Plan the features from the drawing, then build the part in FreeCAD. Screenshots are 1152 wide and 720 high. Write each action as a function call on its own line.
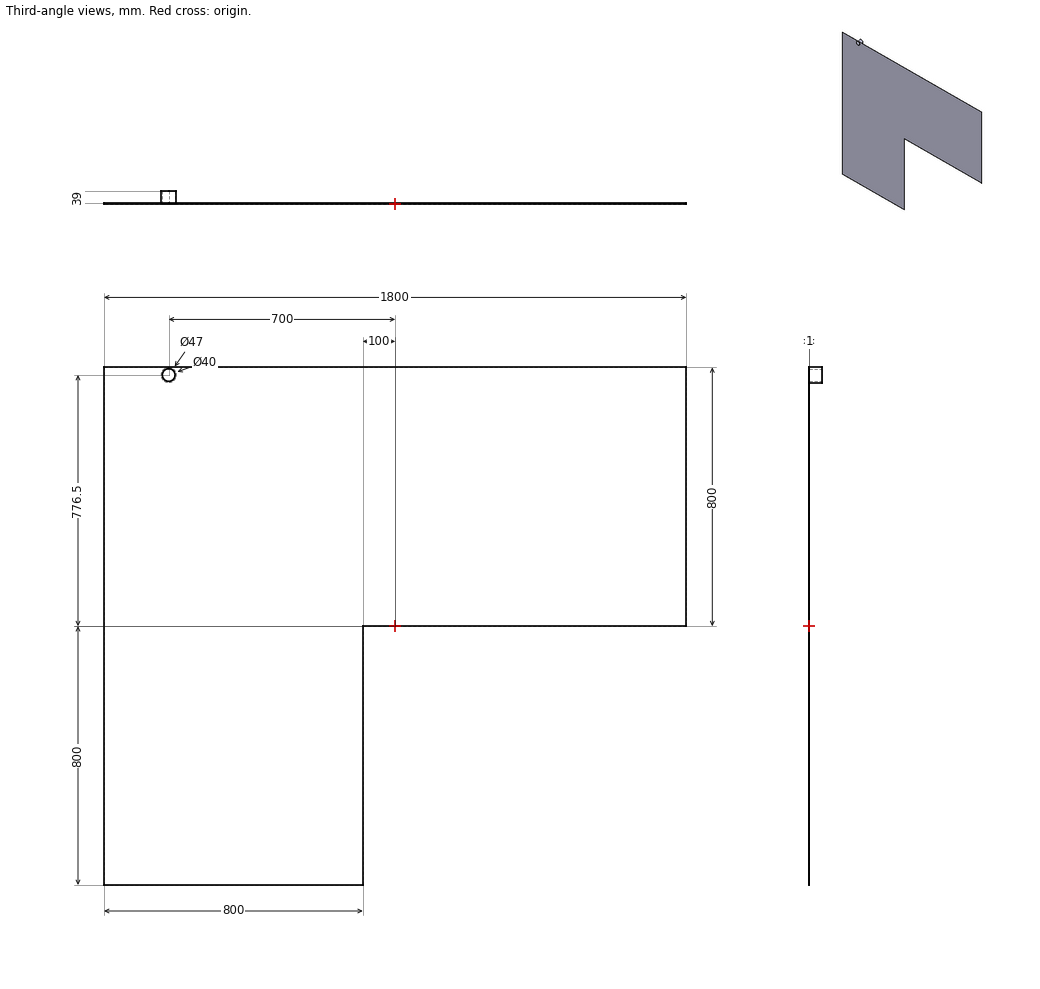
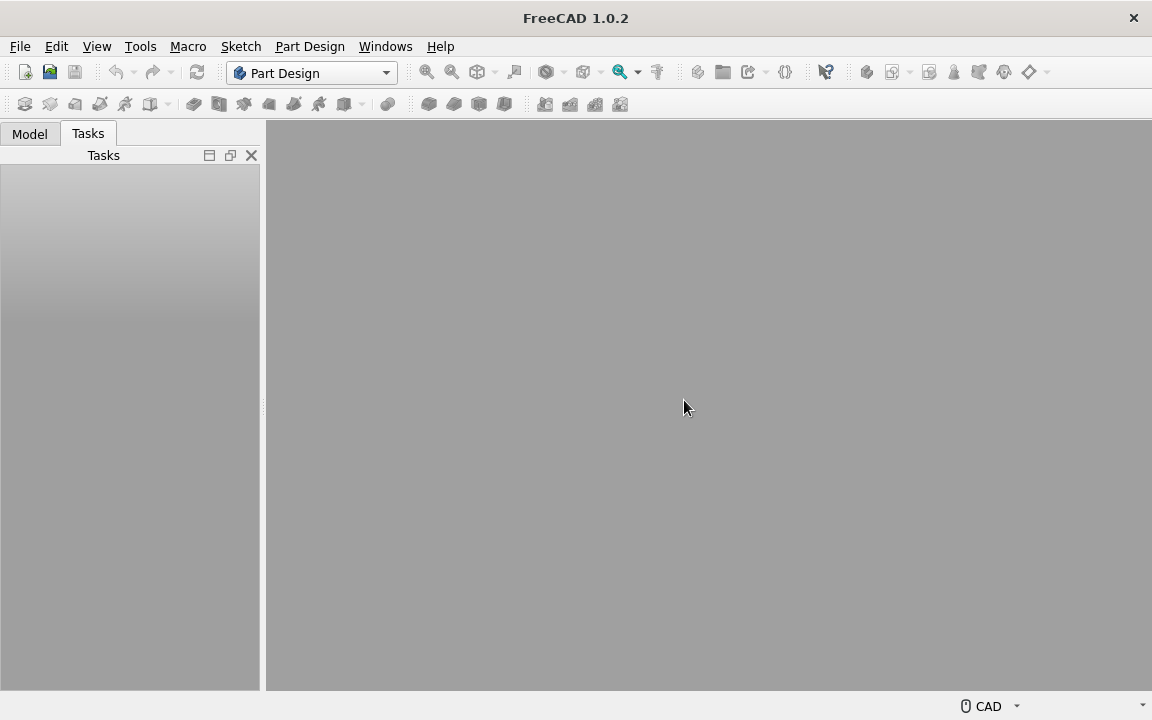
click(25, 72)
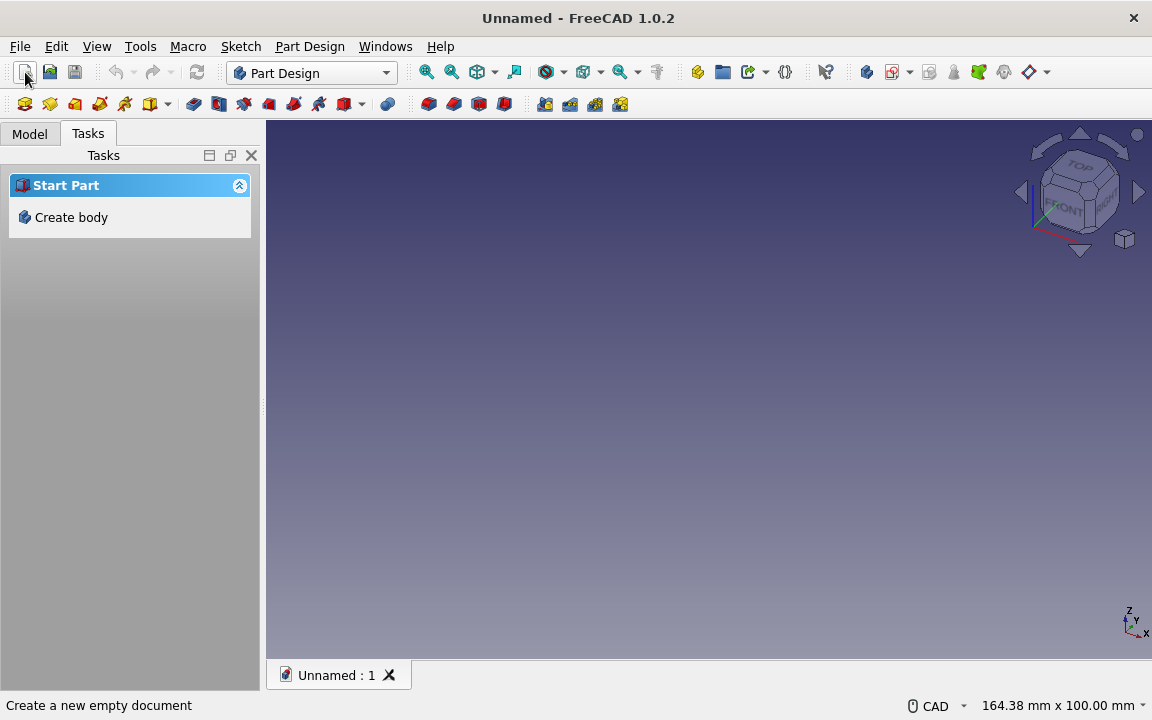
click(892, 72)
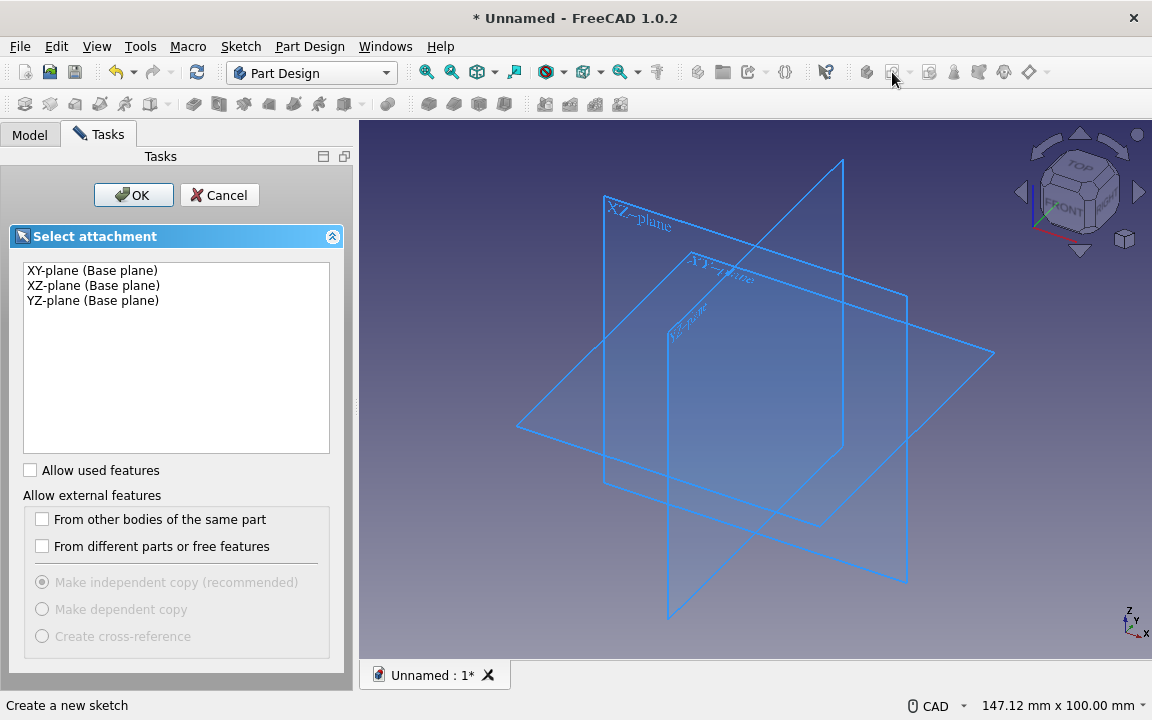
click(84, 286)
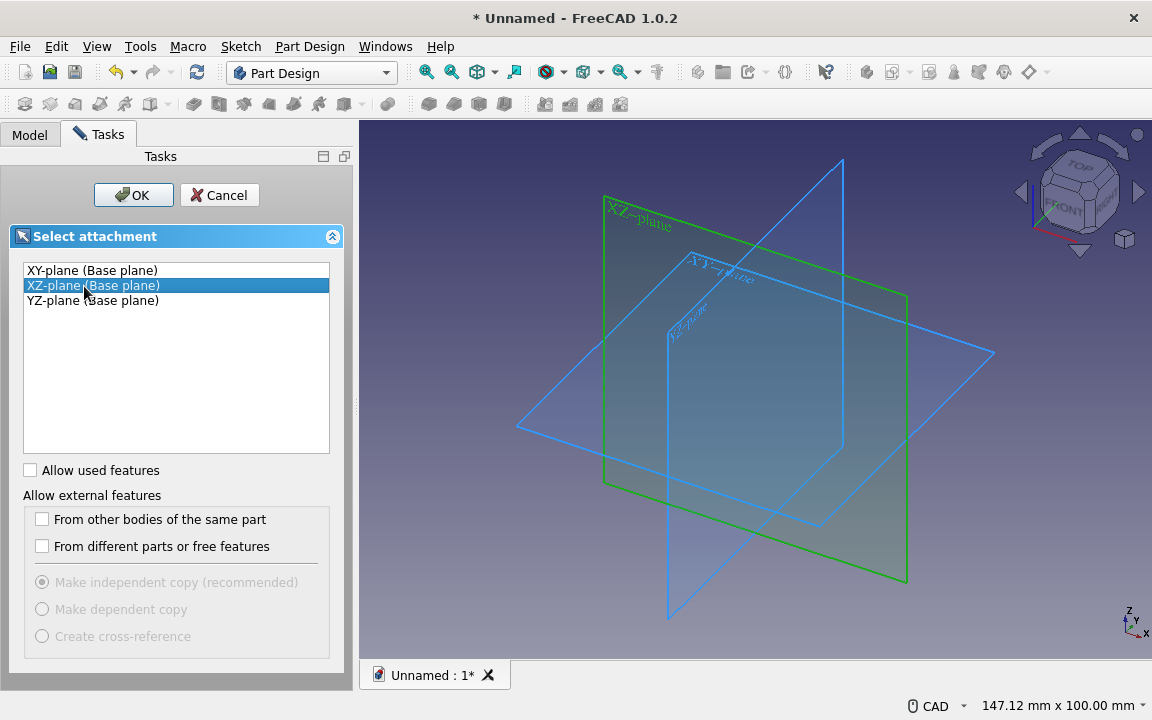
click(134, 195)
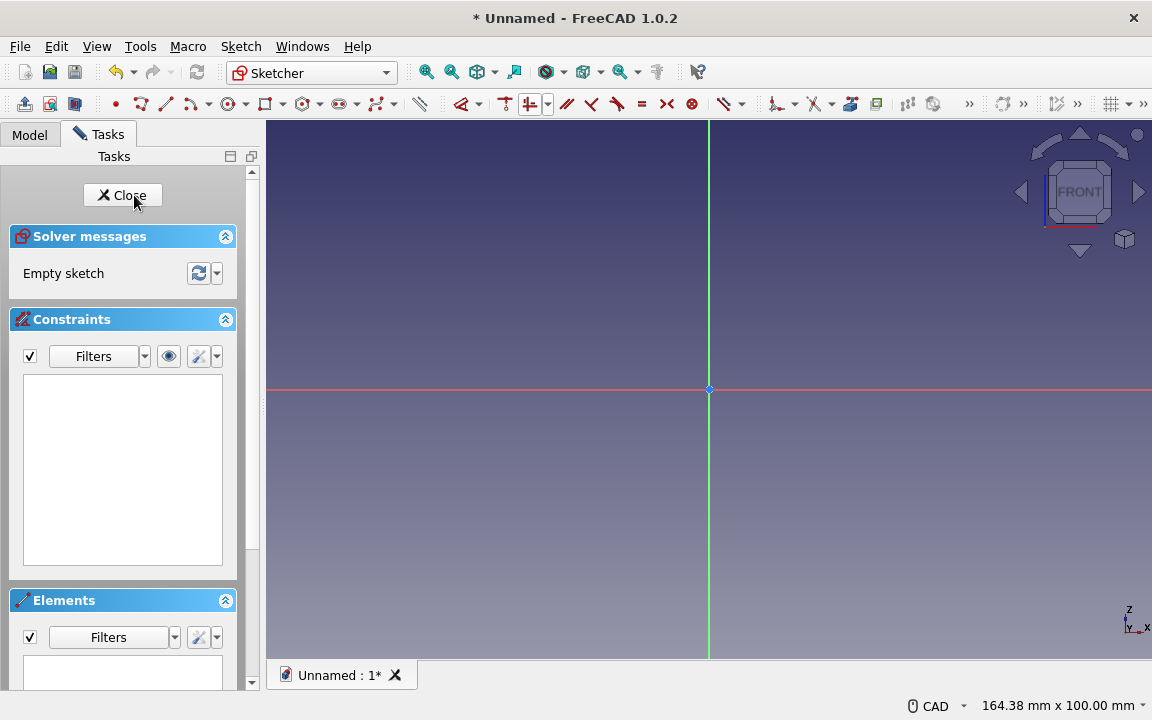
scroll(637, 390, down, 15)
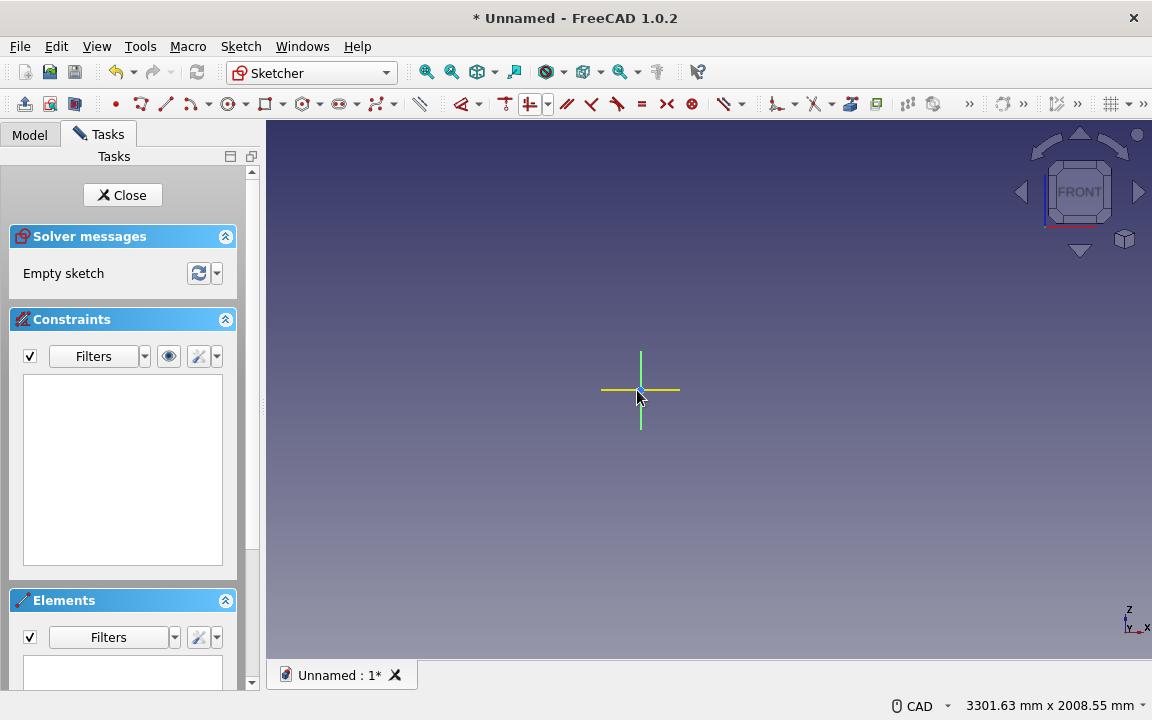
click(141, 104)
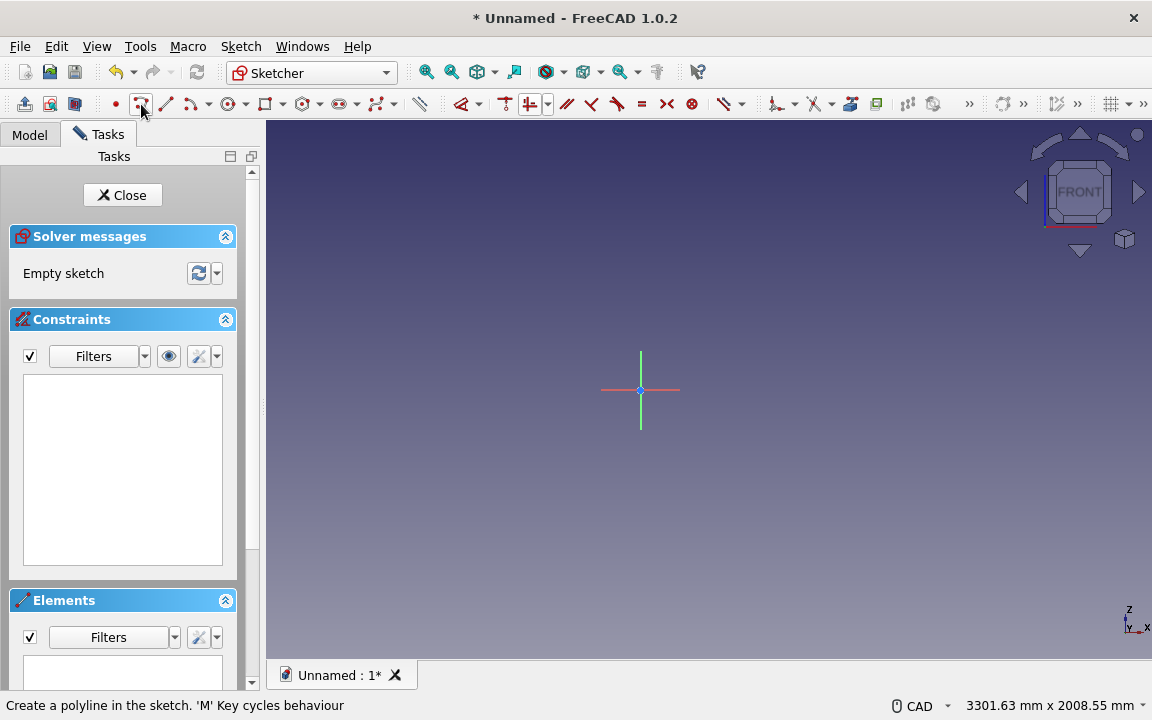
click(614, 390)
click(614, 605)
click(399, 605)
click(399, 176)
click(883, 176)
click(883, 381)
click(614, 390)
key(Escape)
key(Escape)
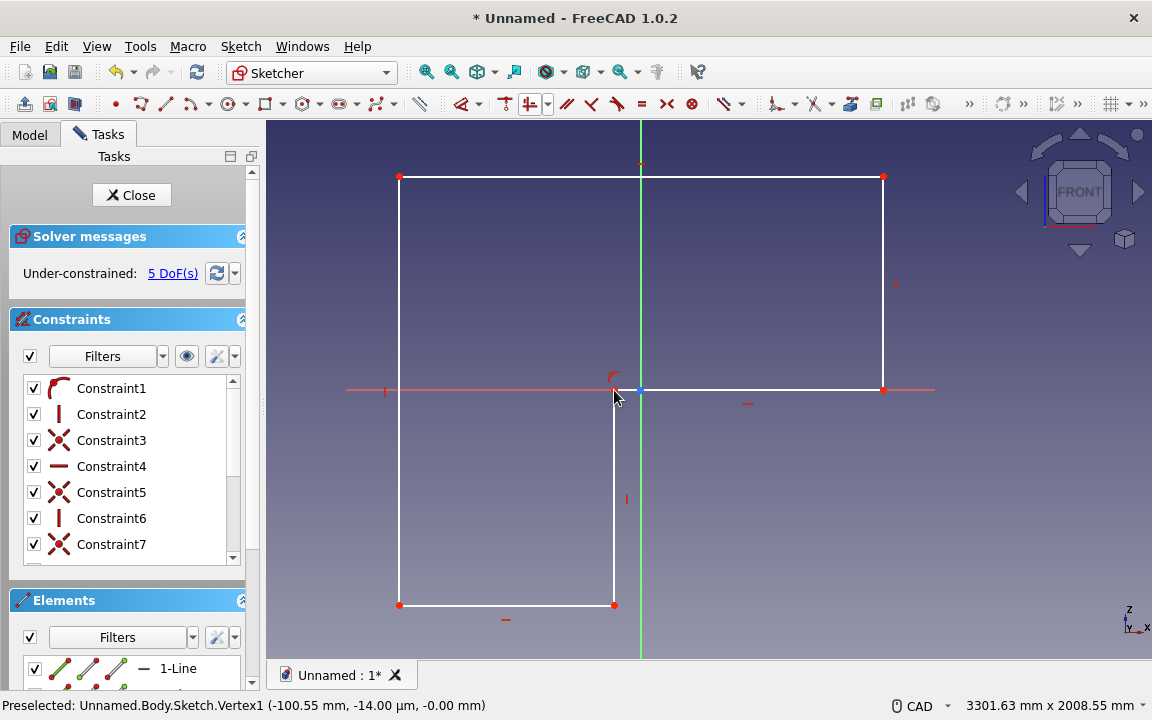
click(614, 455)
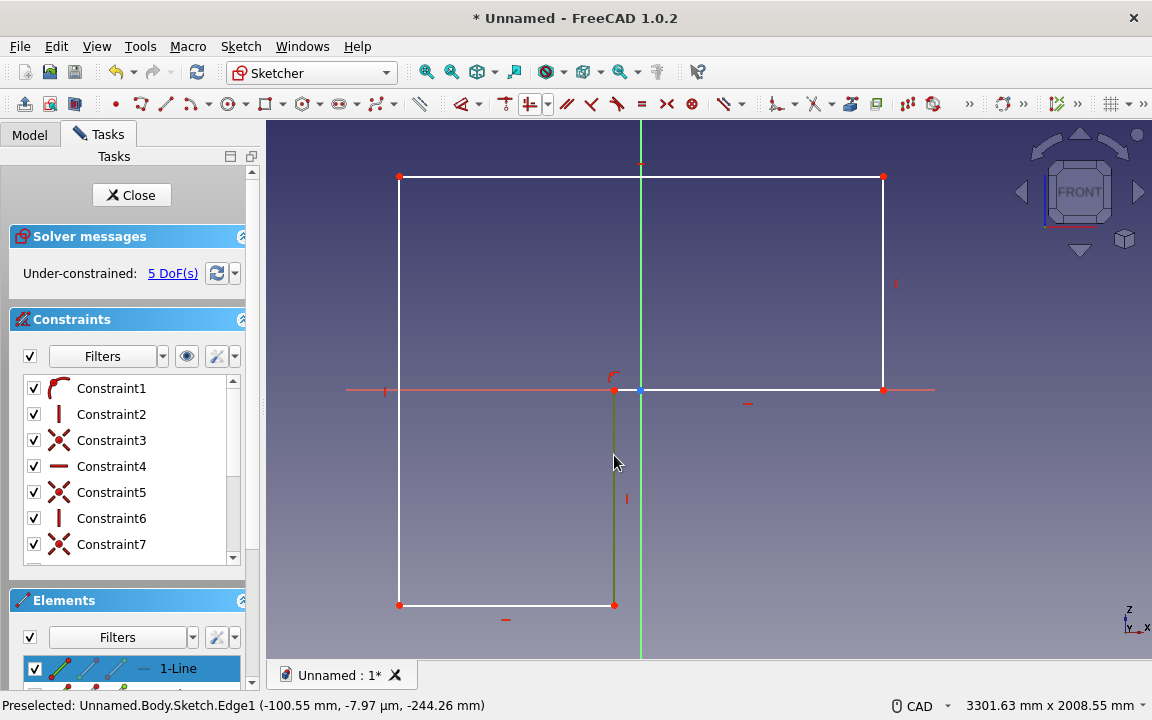
key(i)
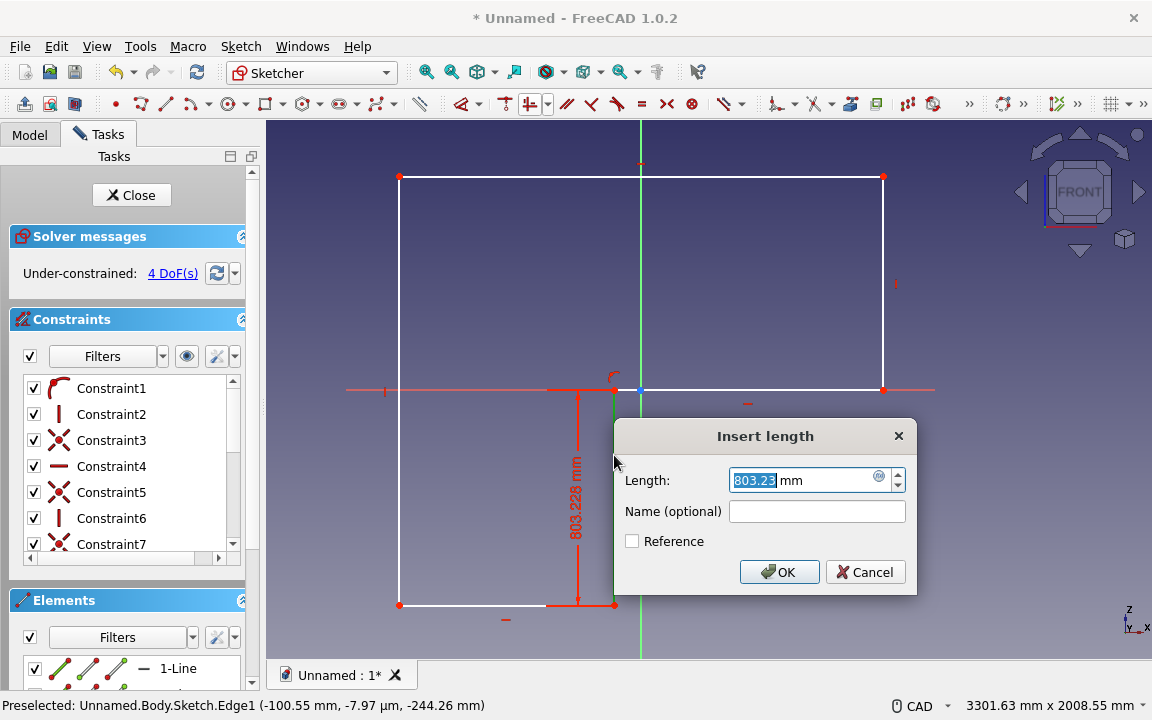
text(800)
key(Return)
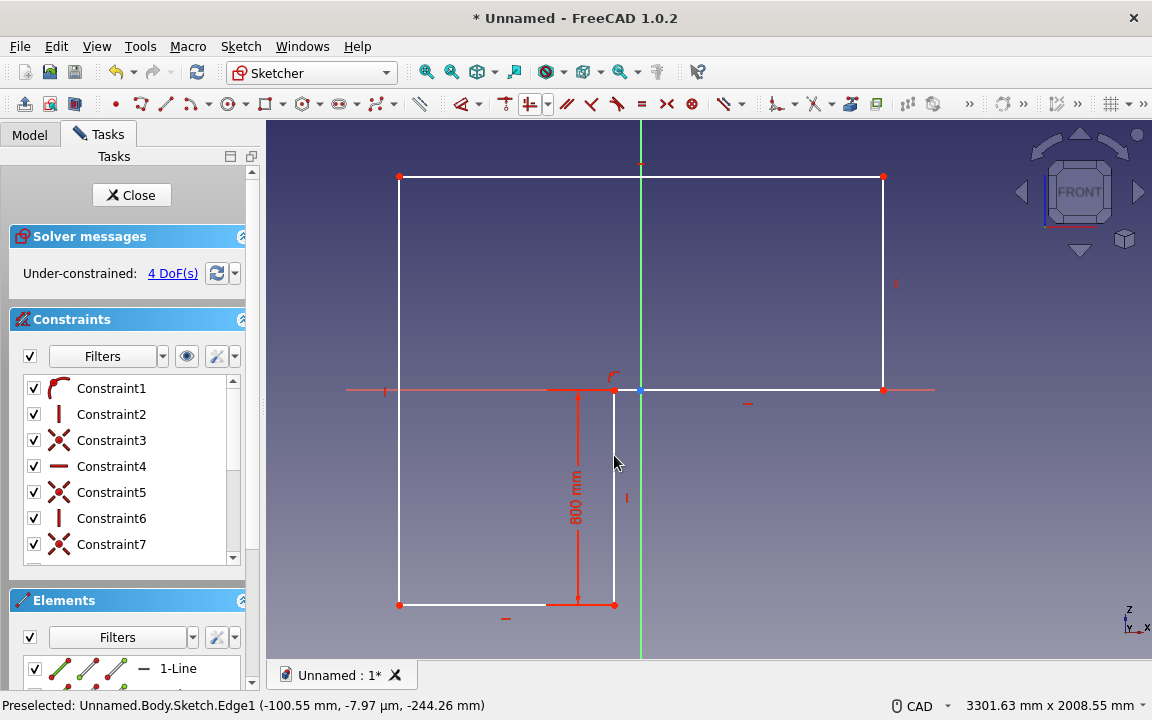
click(550, 605)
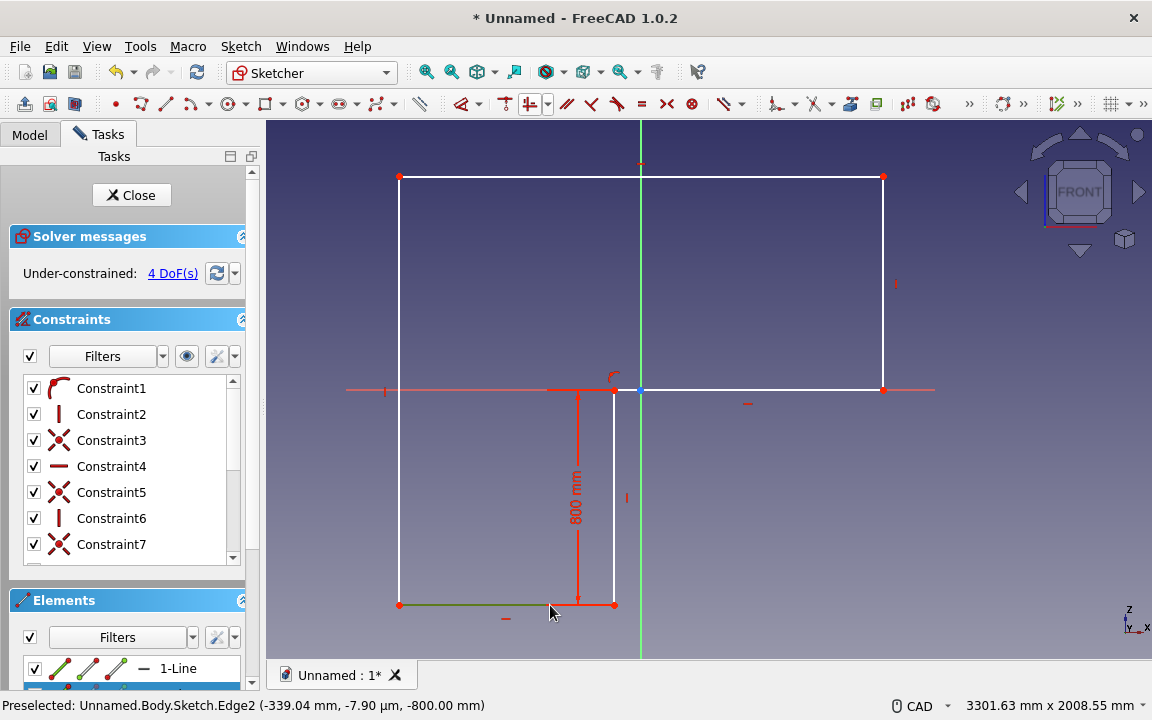
click(478, 104)